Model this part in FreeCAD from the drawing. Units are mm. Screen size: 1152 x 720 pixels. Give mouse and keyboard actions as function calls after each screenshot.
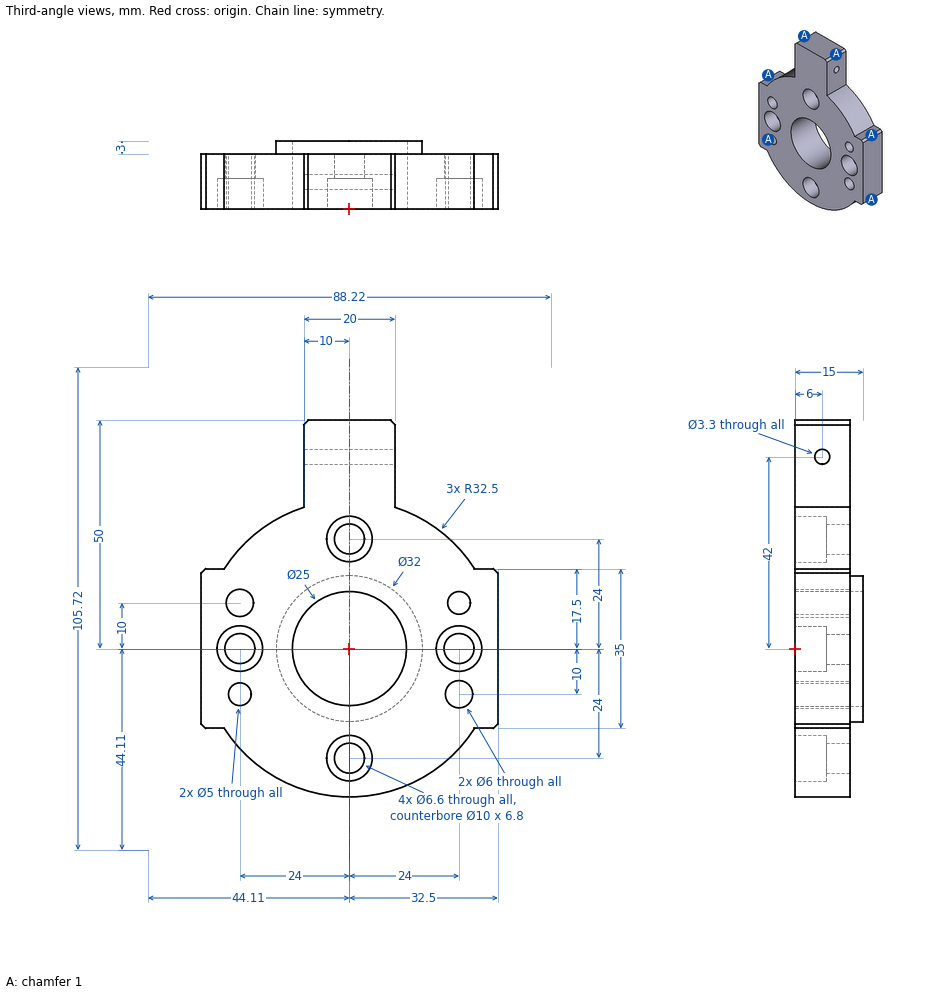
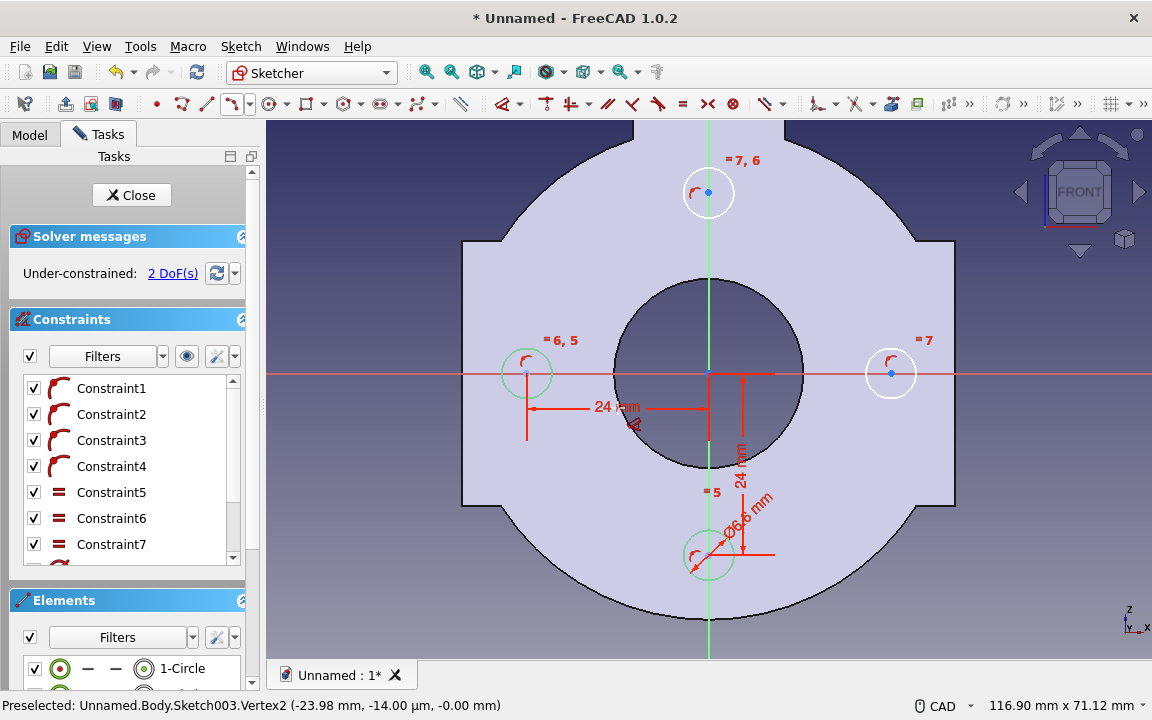
click(709, 193)
click(743, 283)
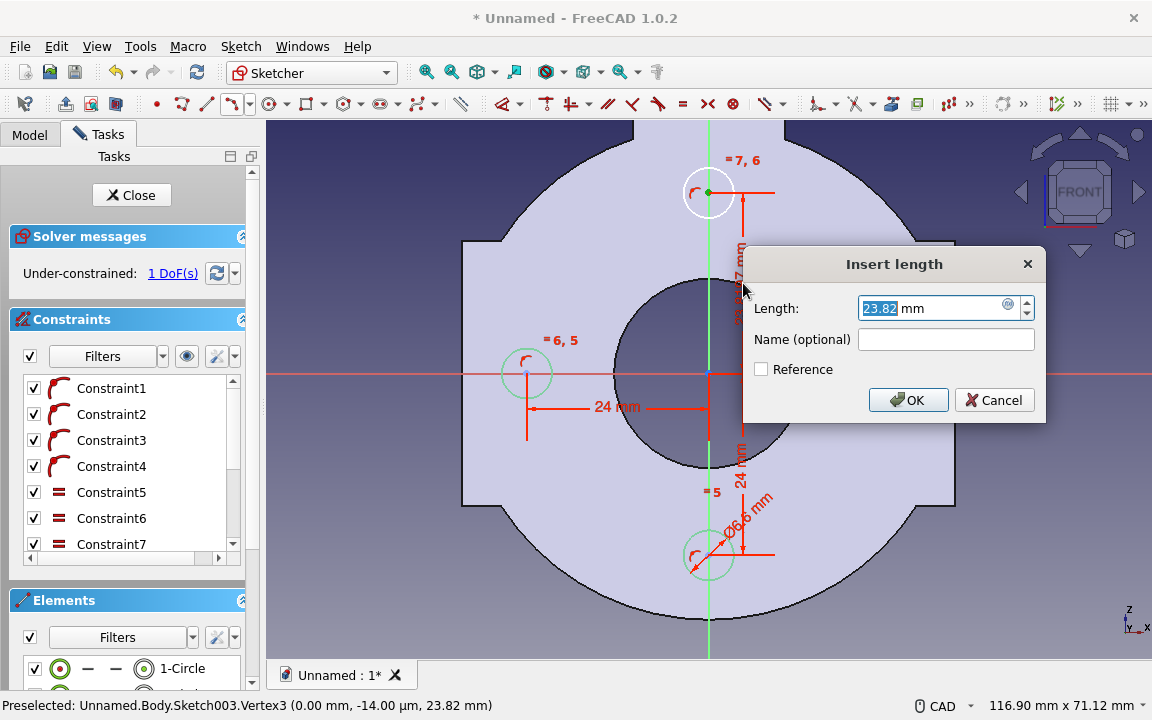
text(24)
key(Return)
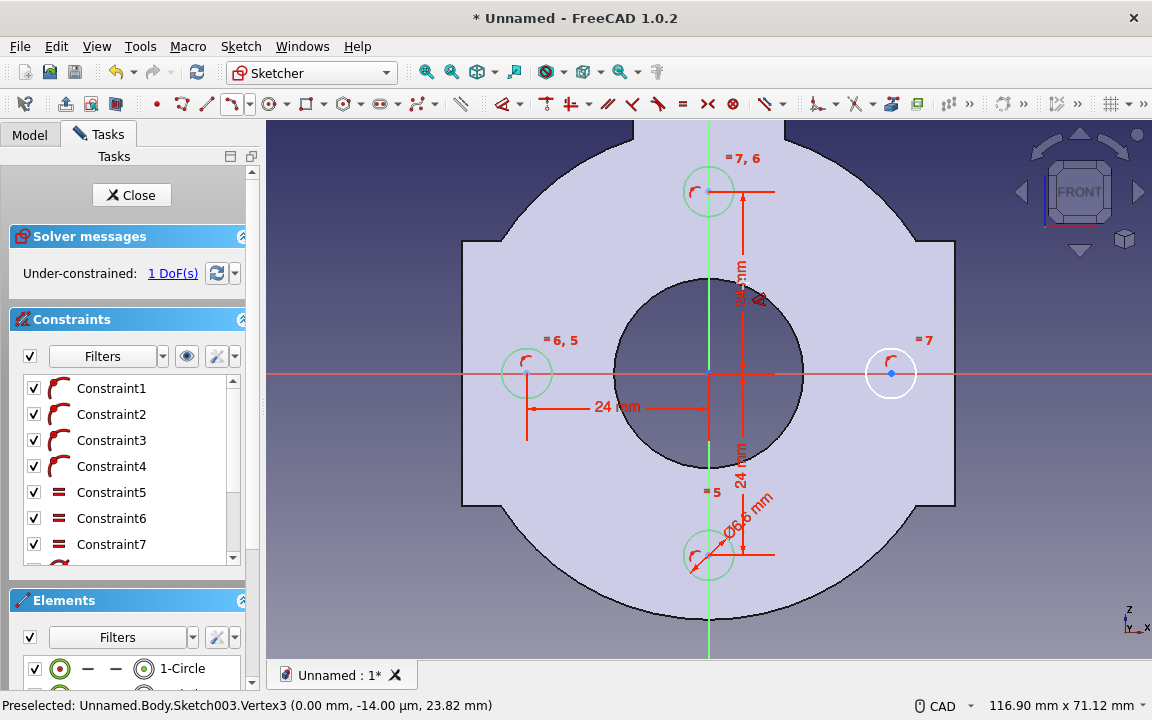
click(891, 374)
click(800, 408)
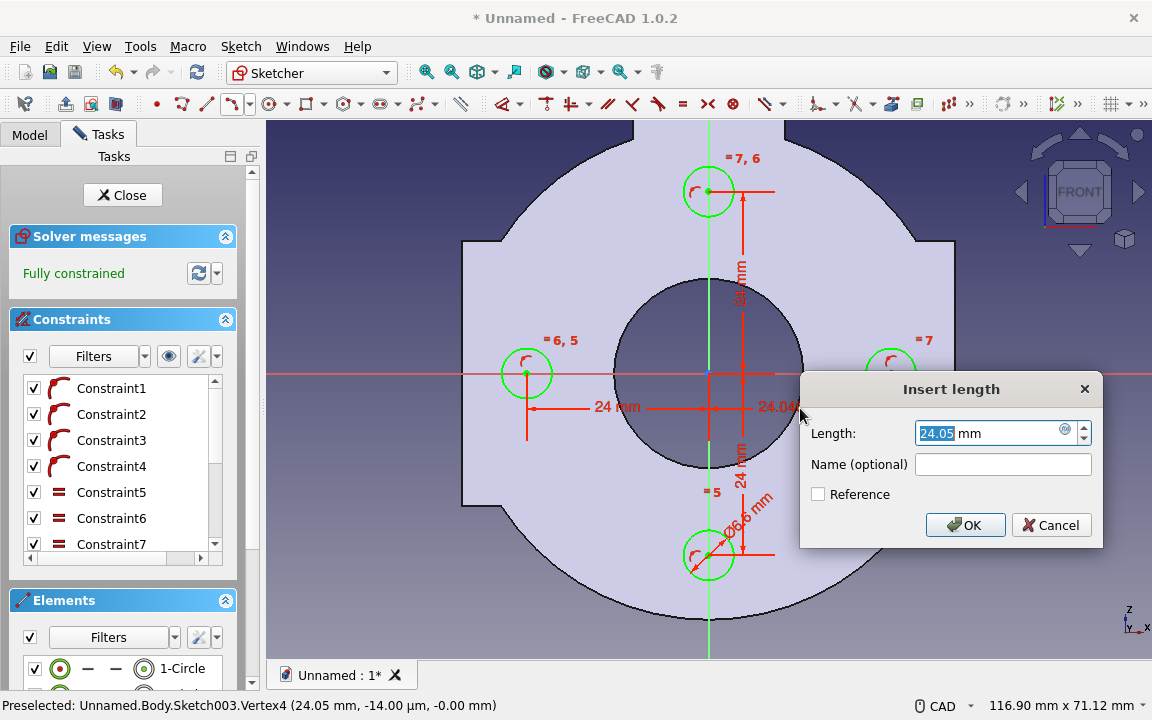
text(24)
key(Return)
key(Escape)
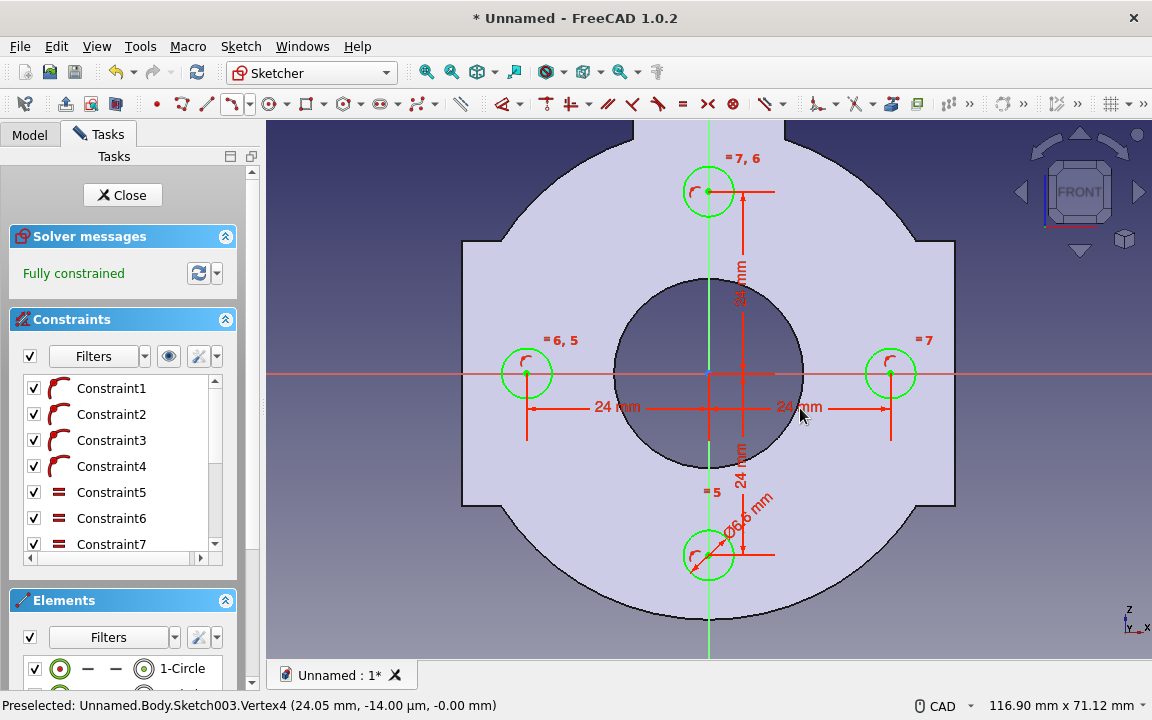
click(123, 195)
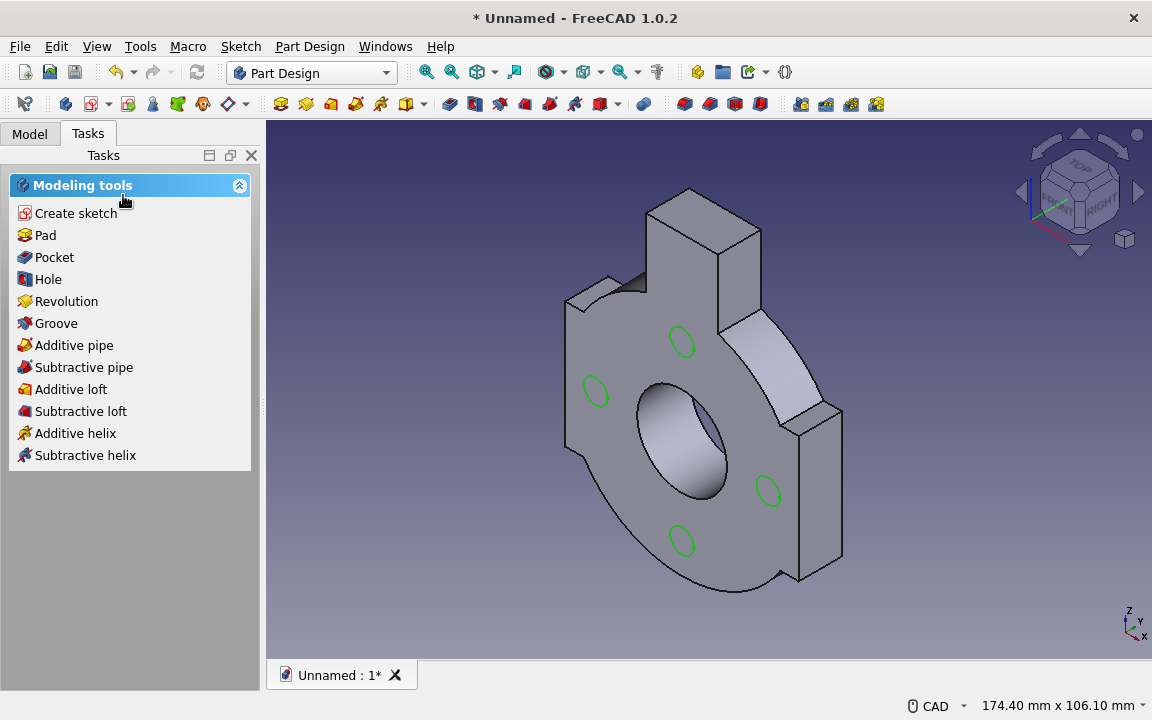
click(475, 104)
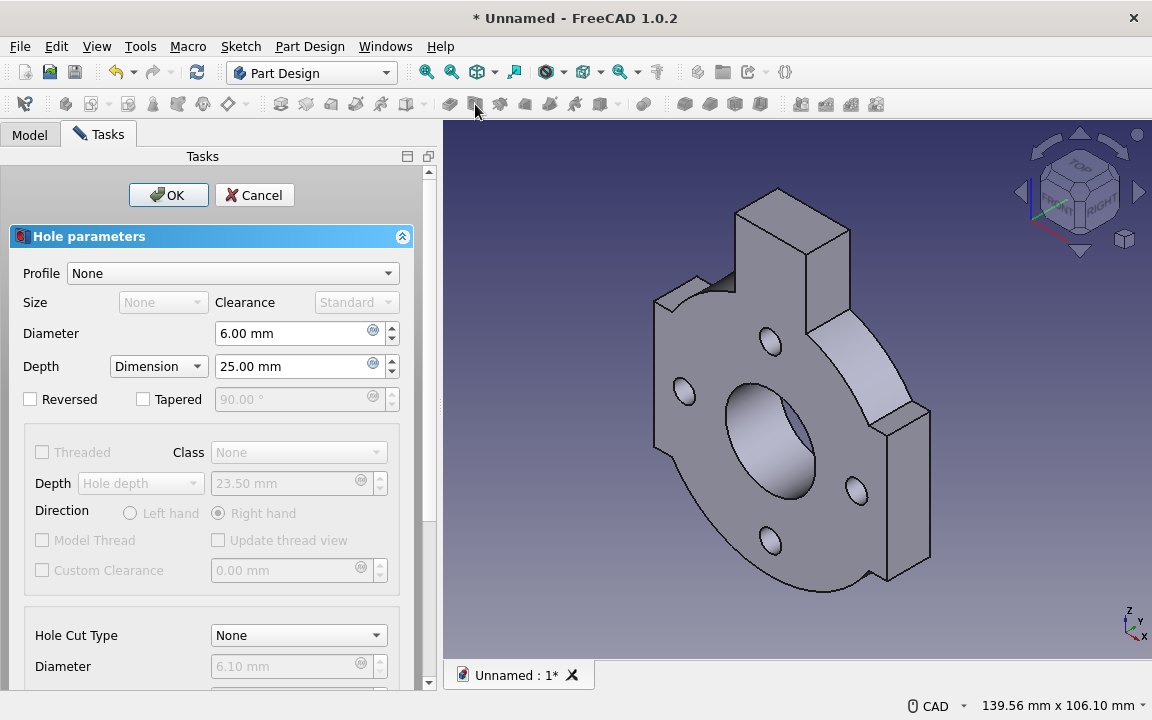
triple_click(300, 334)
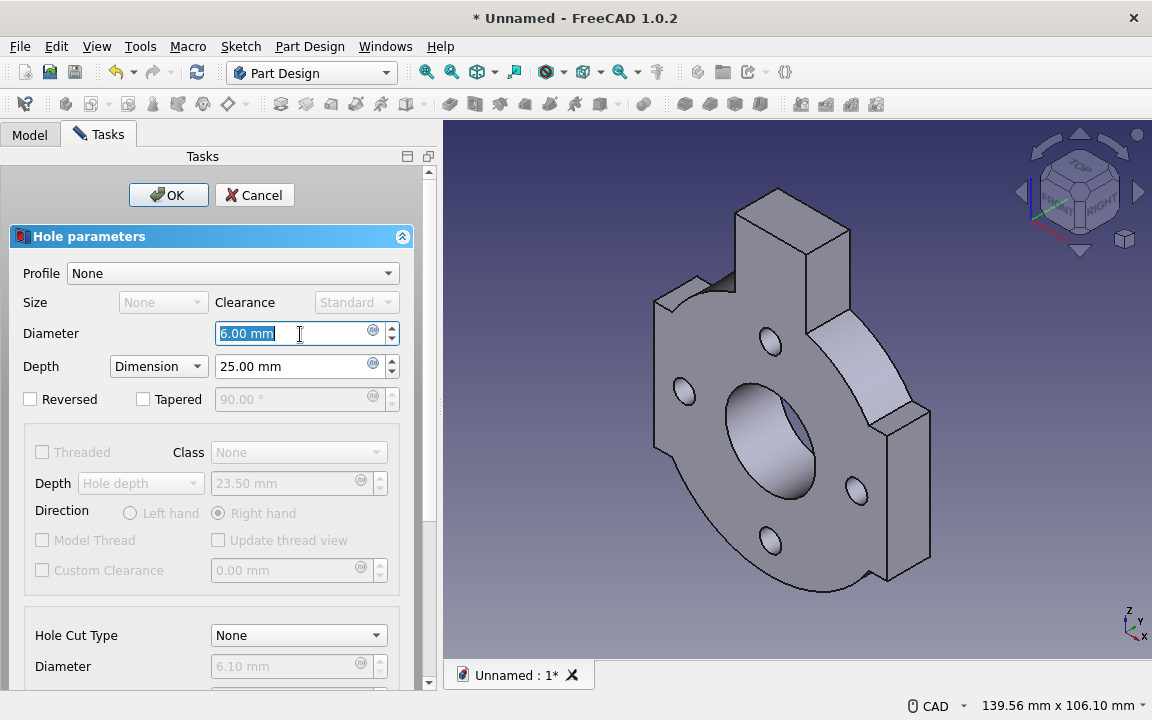
text(6.6)
key(Tab)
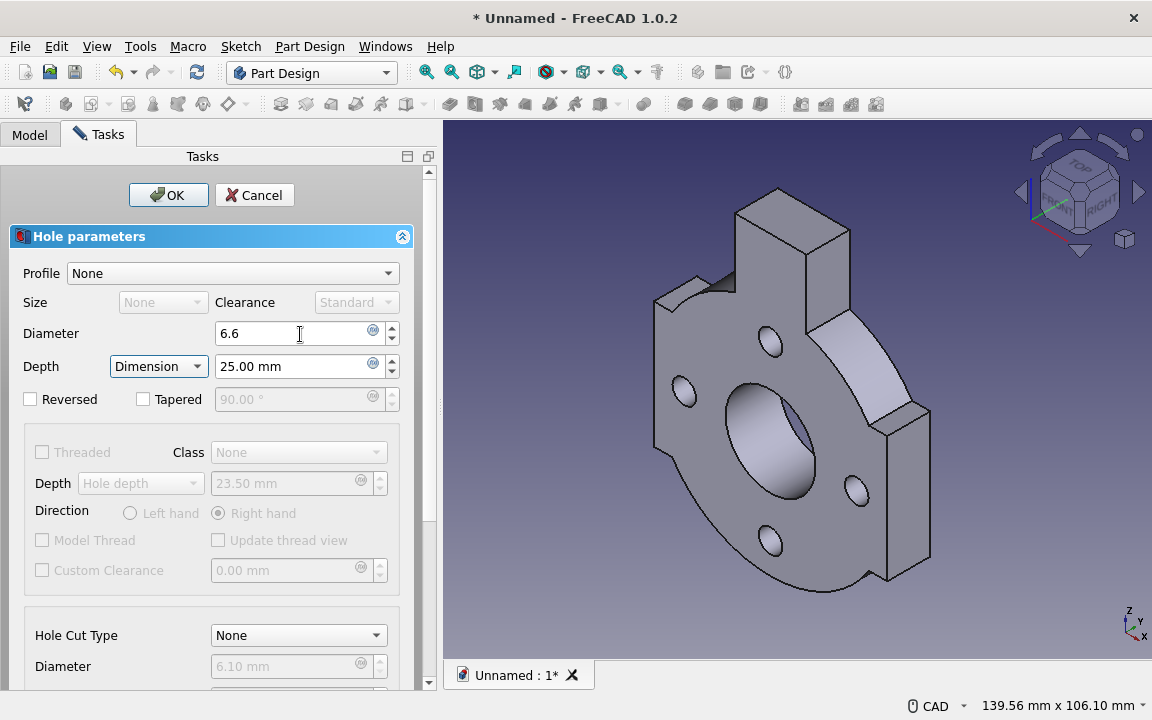
click(160, 366)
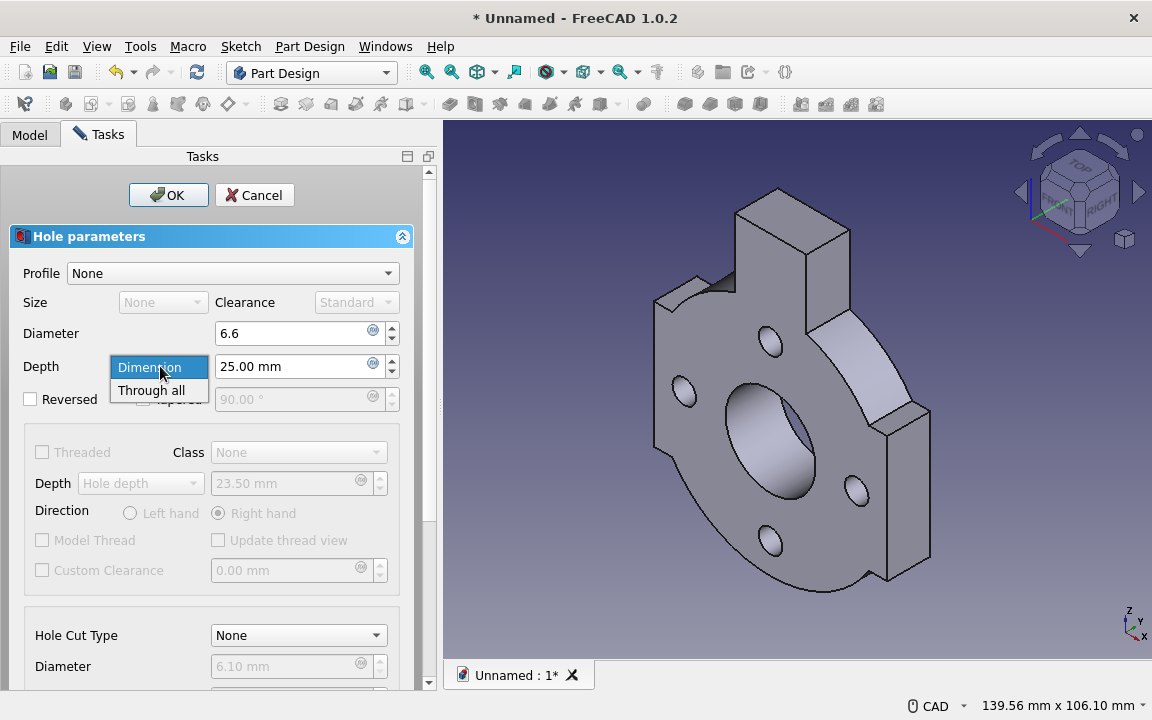
click(158, 390)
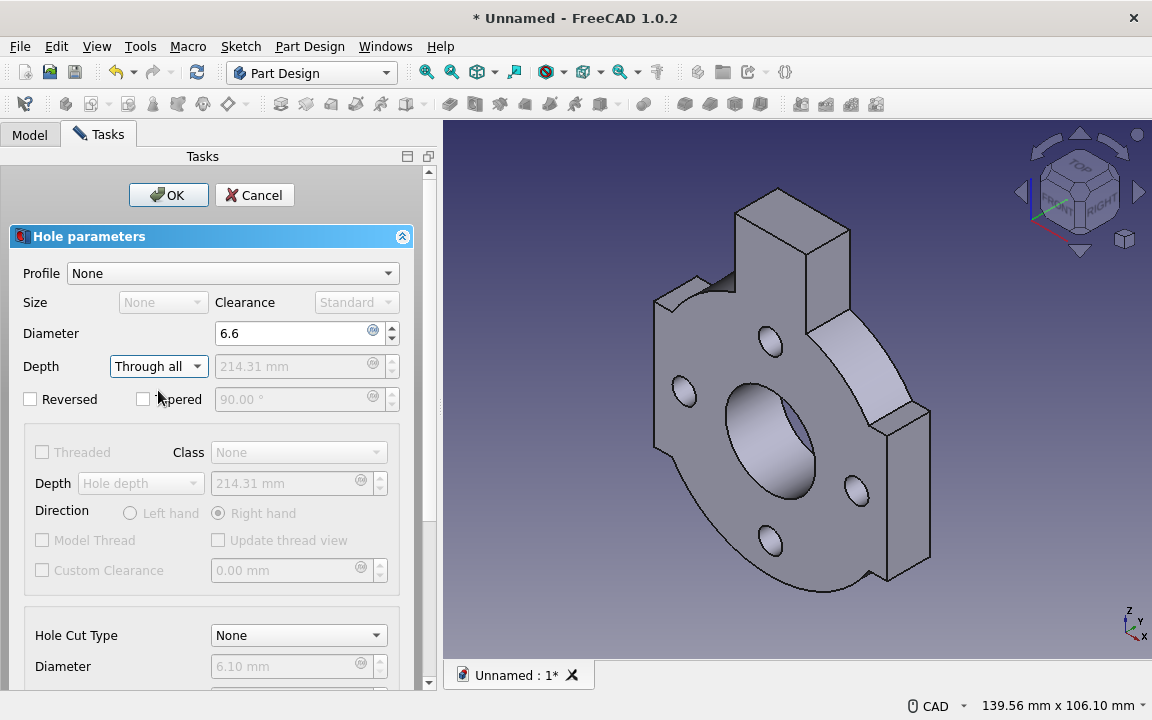
click(300, 636)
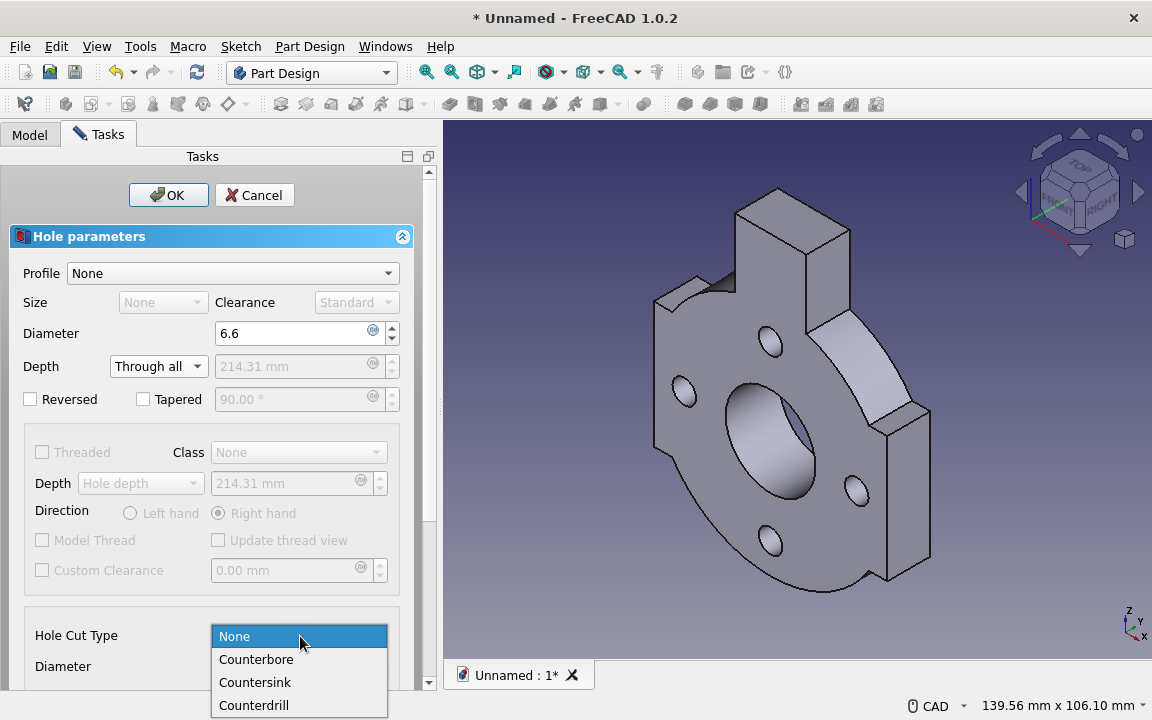
click(298, 660)